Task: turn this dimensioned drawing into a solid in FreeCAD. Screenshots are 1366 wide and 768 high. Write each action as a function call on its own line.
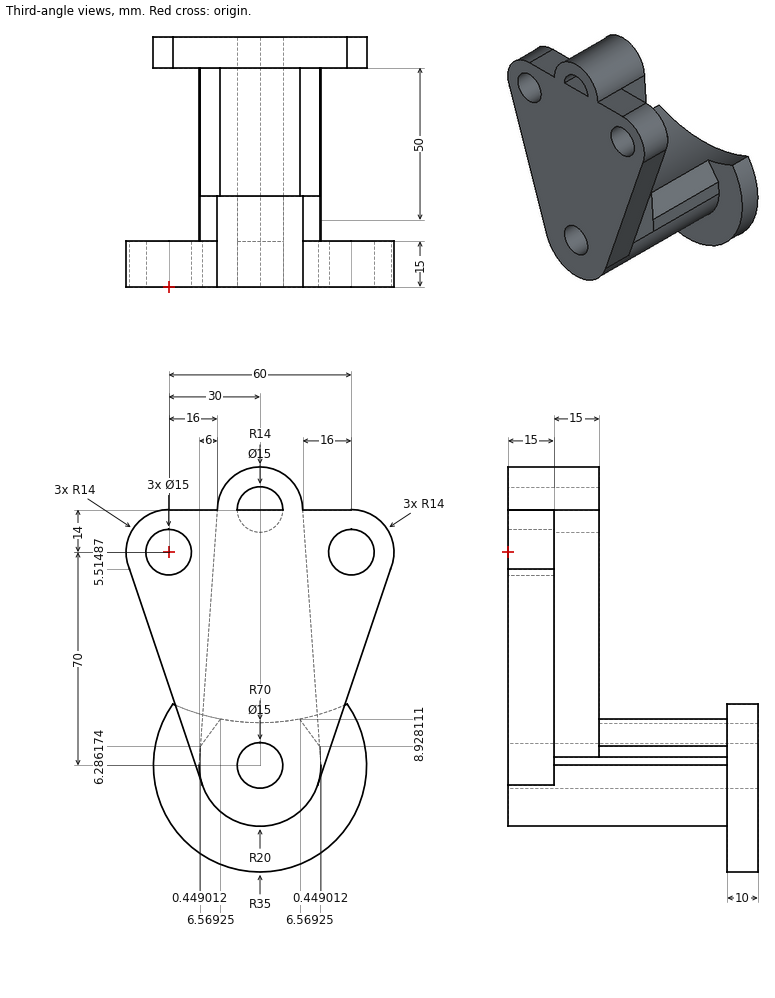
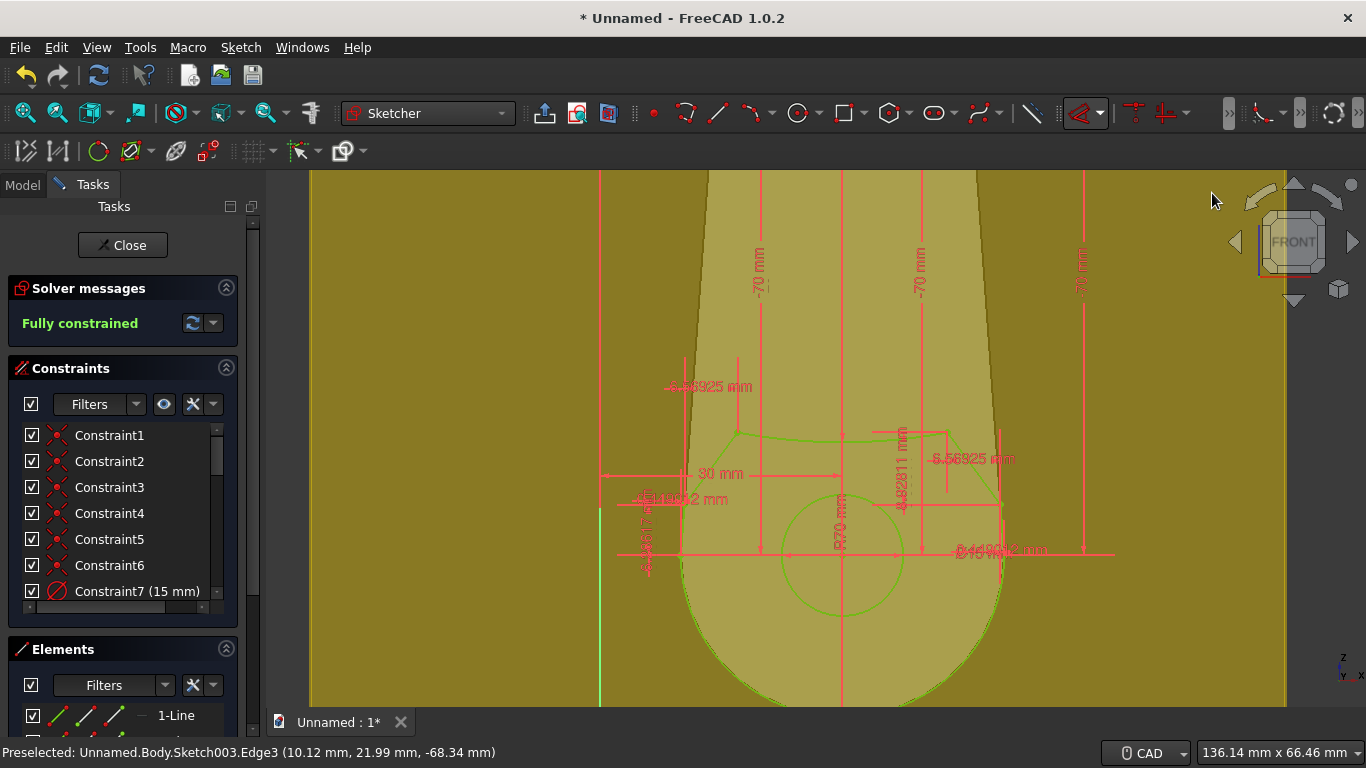
click(123, 245)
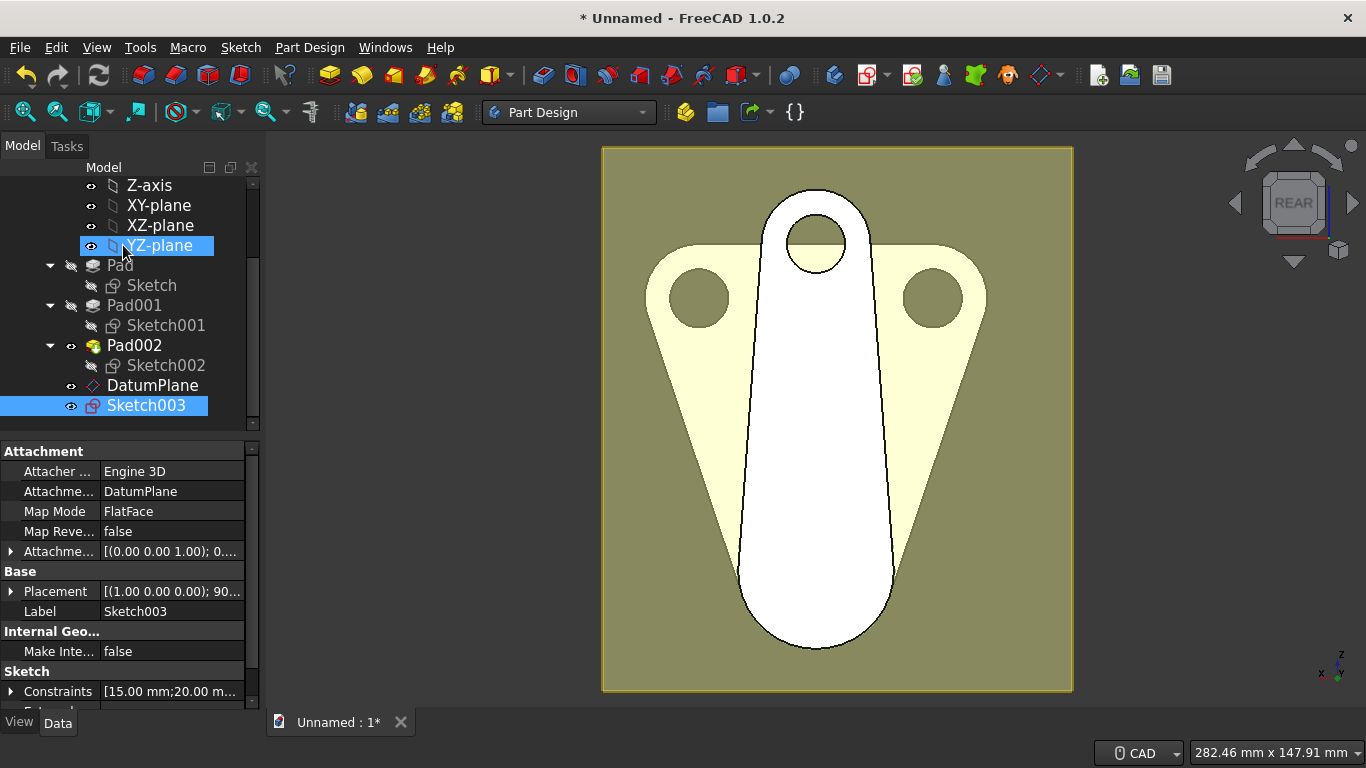
click(330, 76)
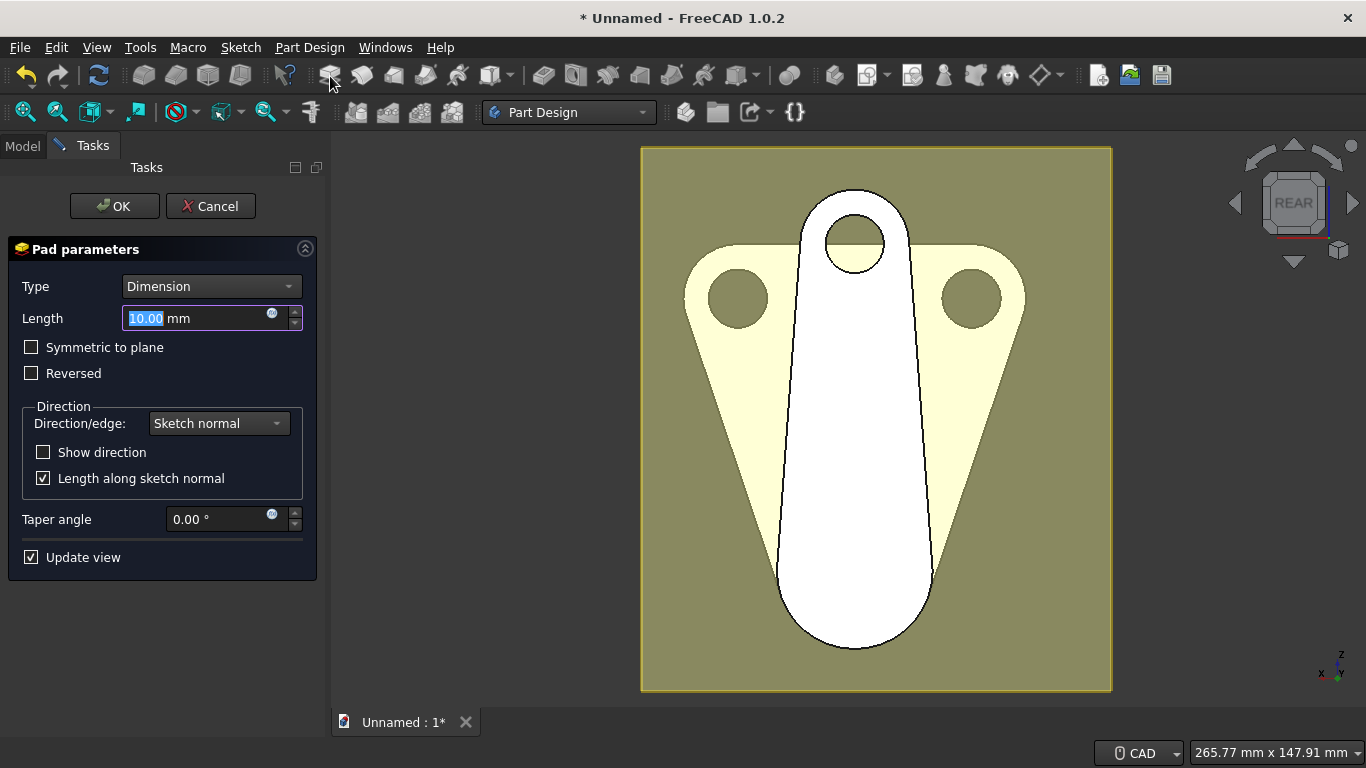
text(50)
key(Tab)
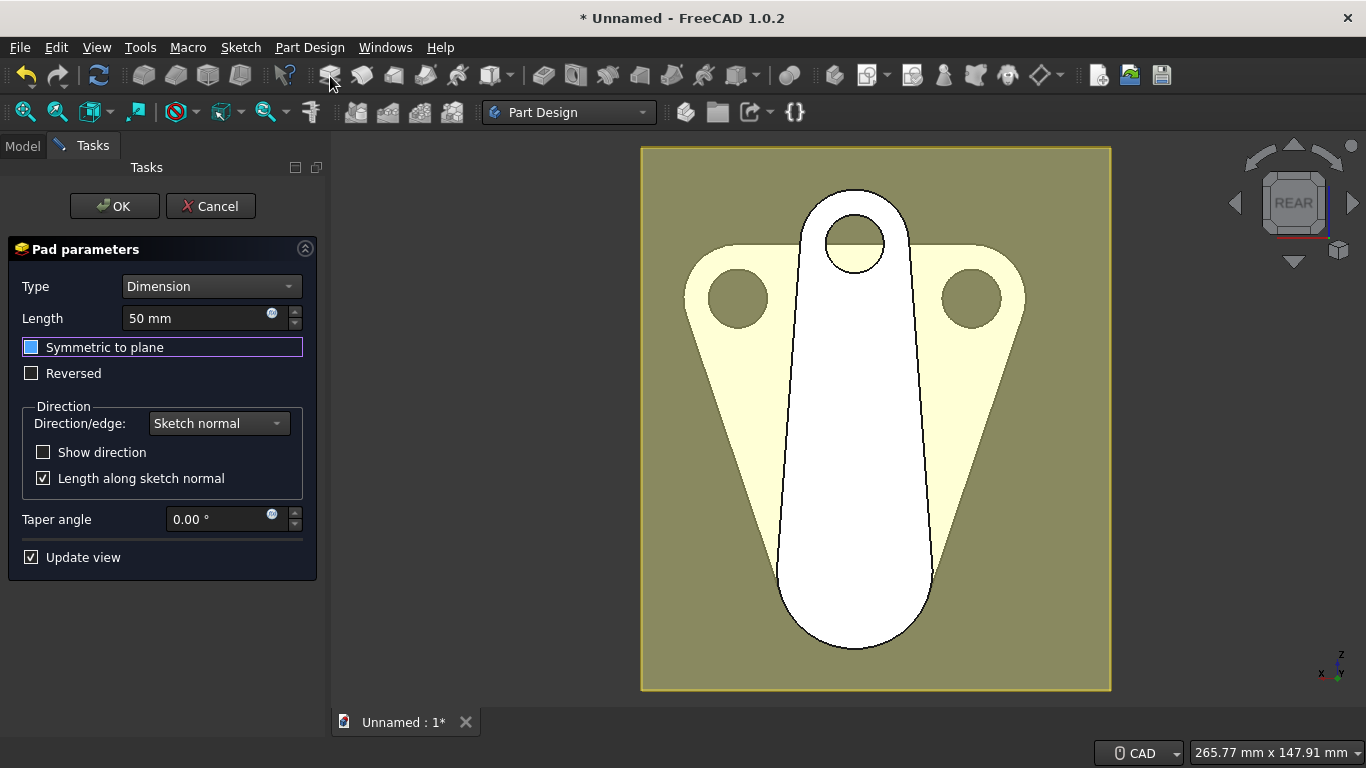
click(30, 373)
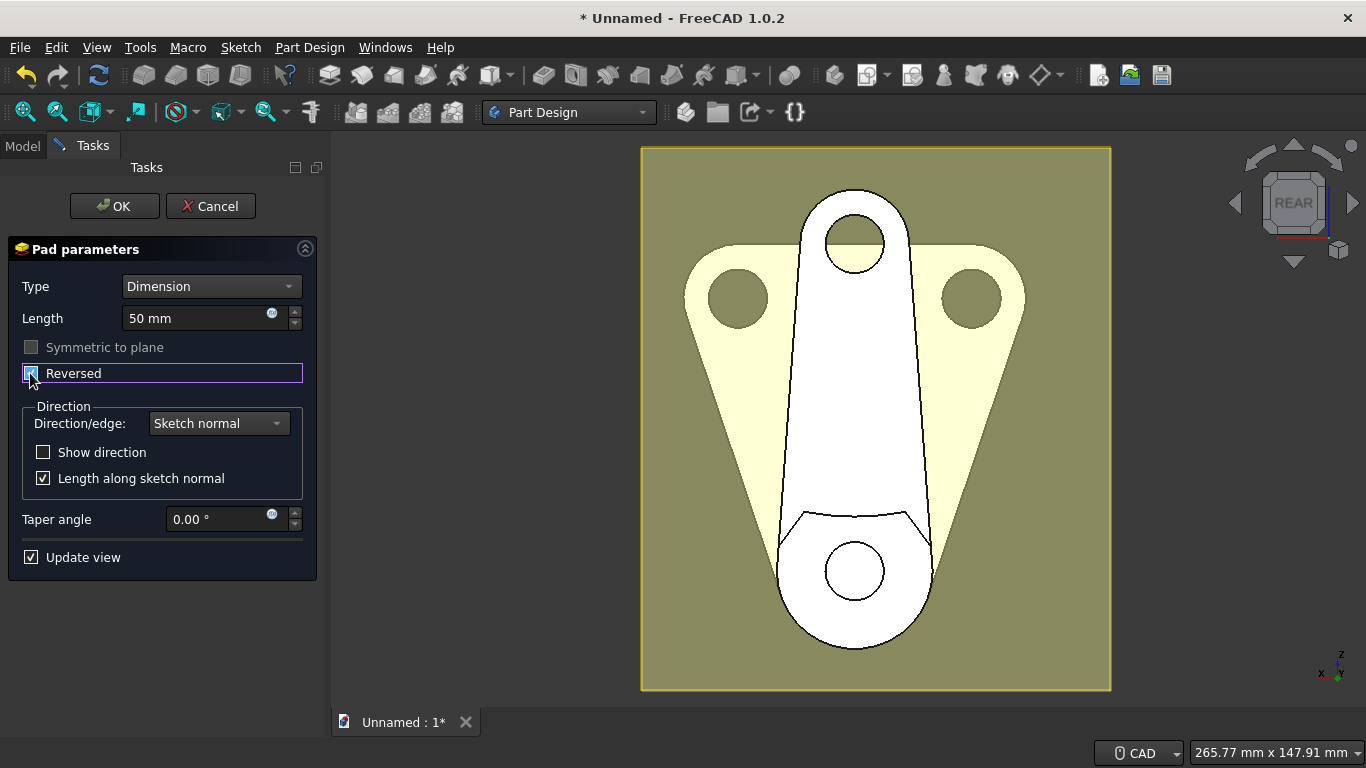
click(115, 206)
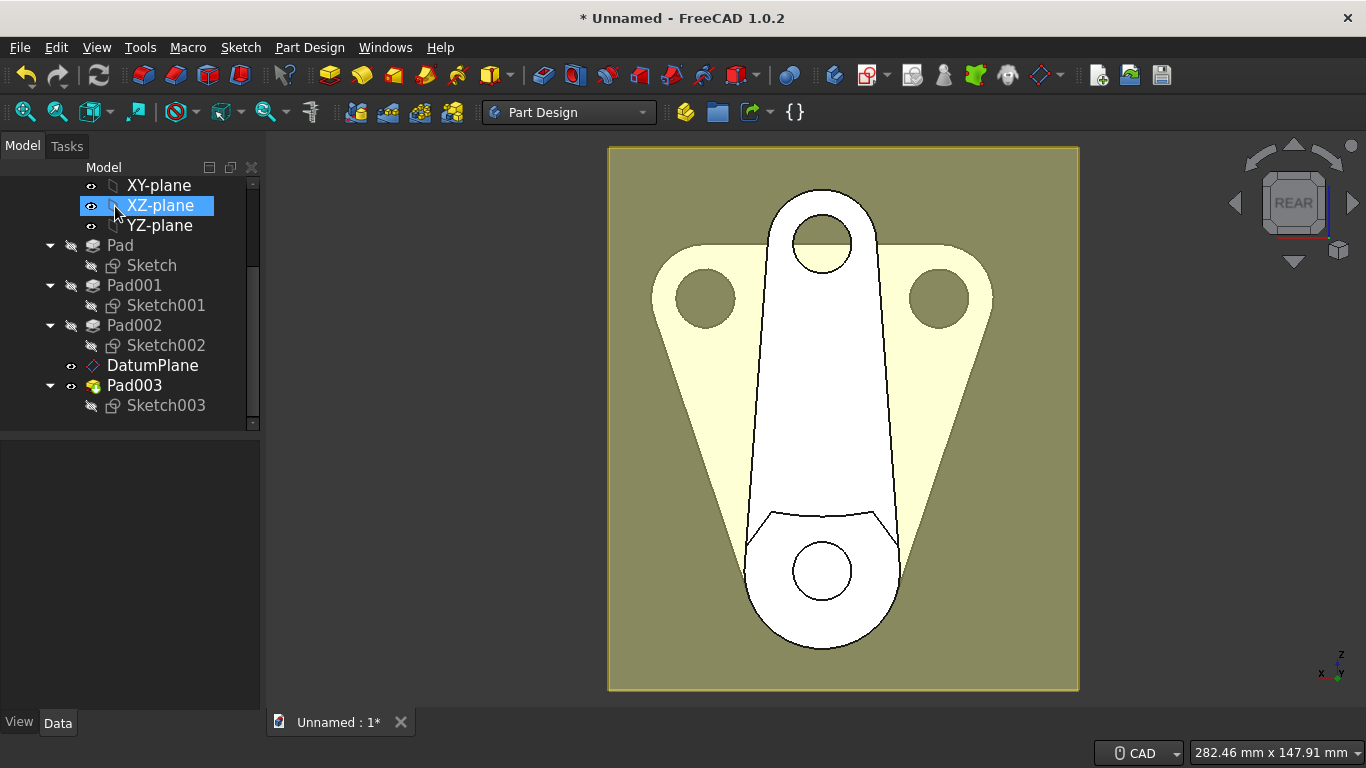
click(116, 366)
key(space)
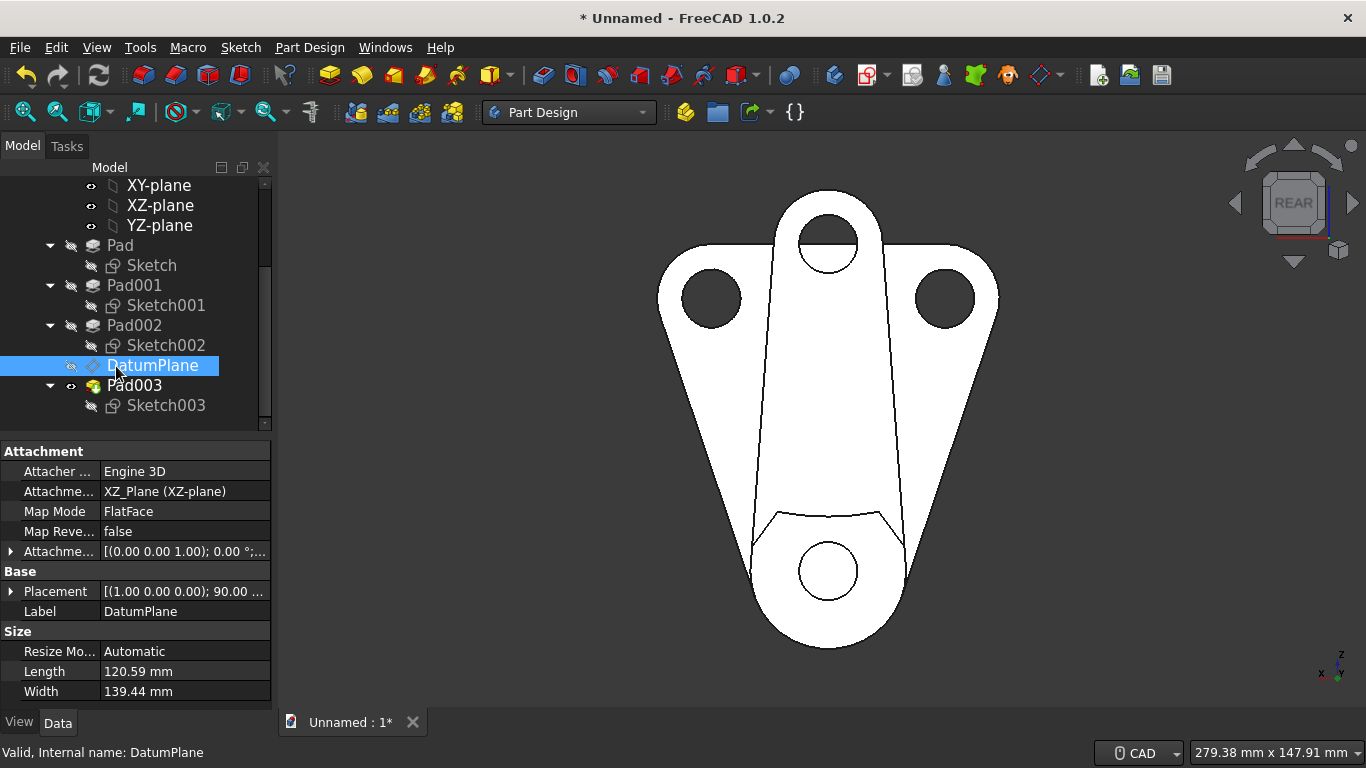
click(806, 619)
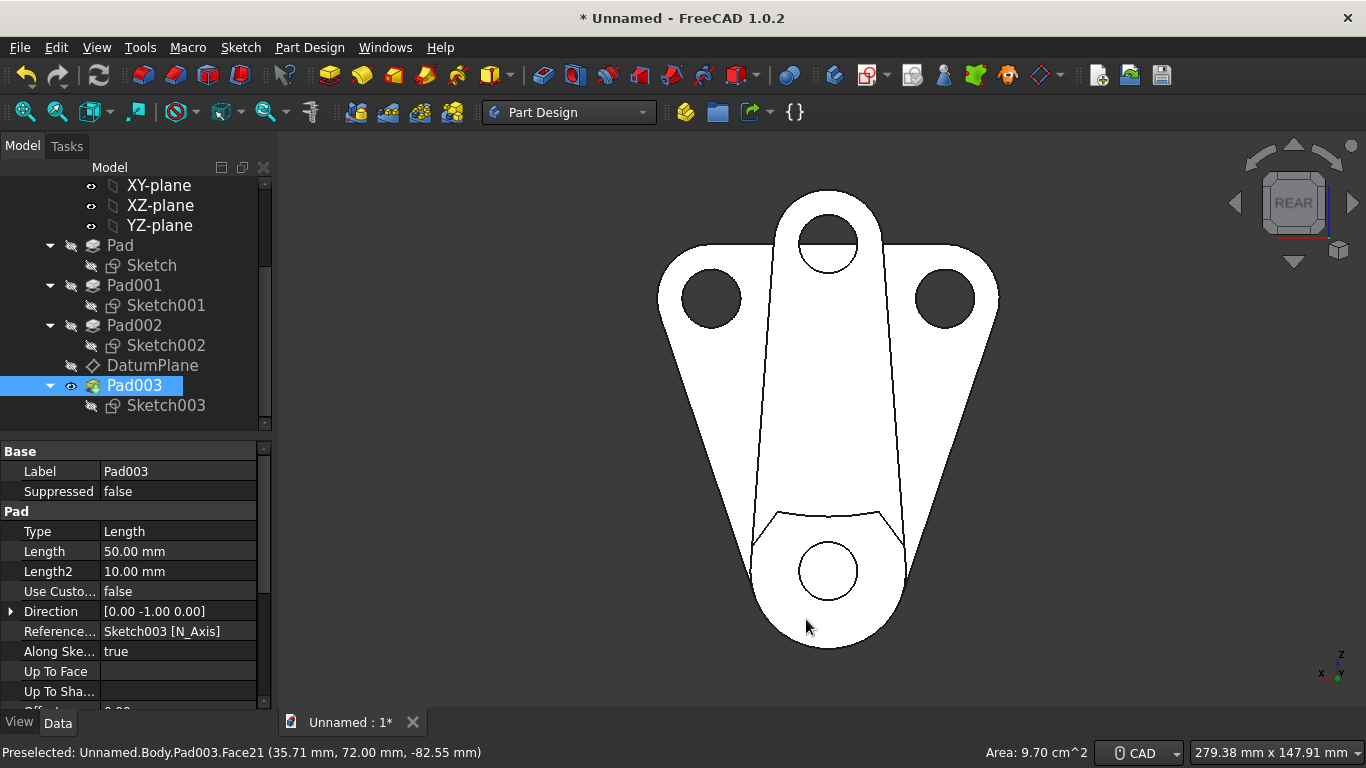
click(868, 76)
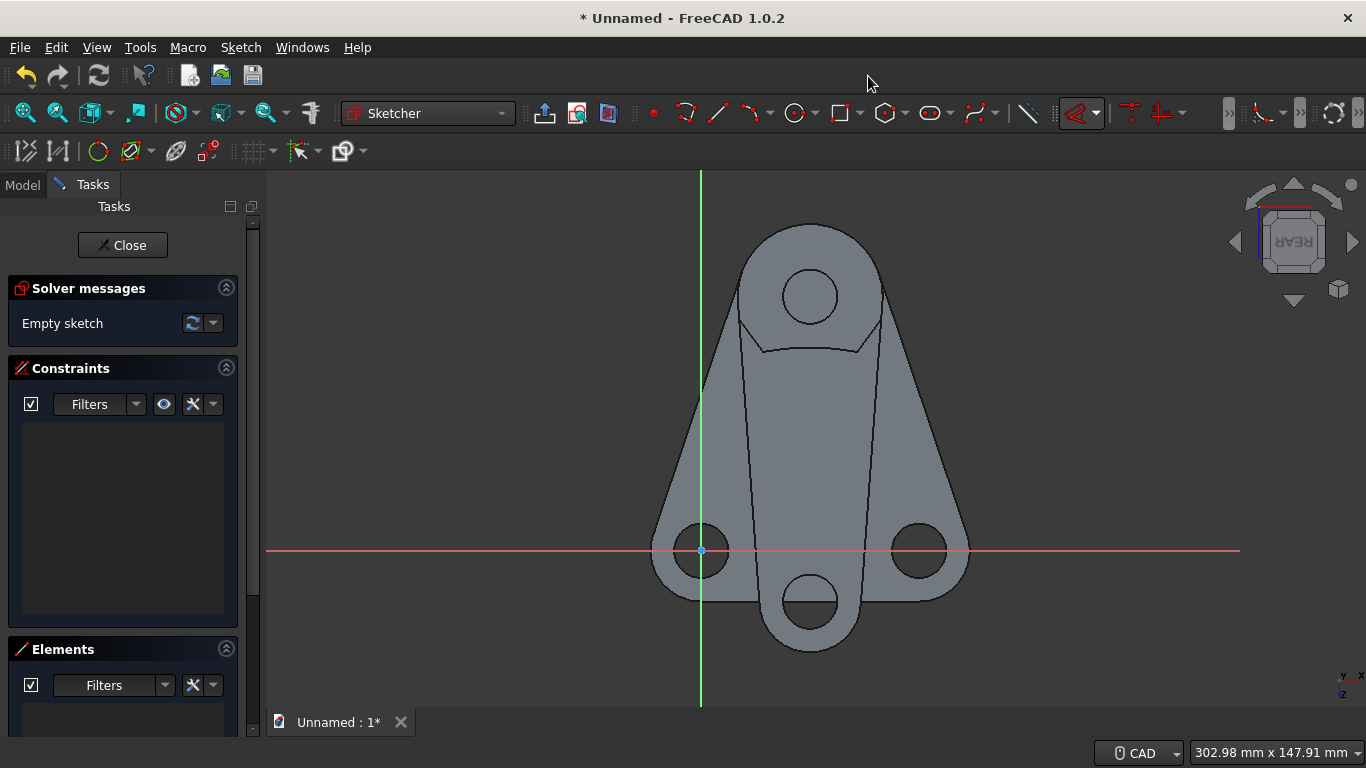
scroll(476, 679, down, 1)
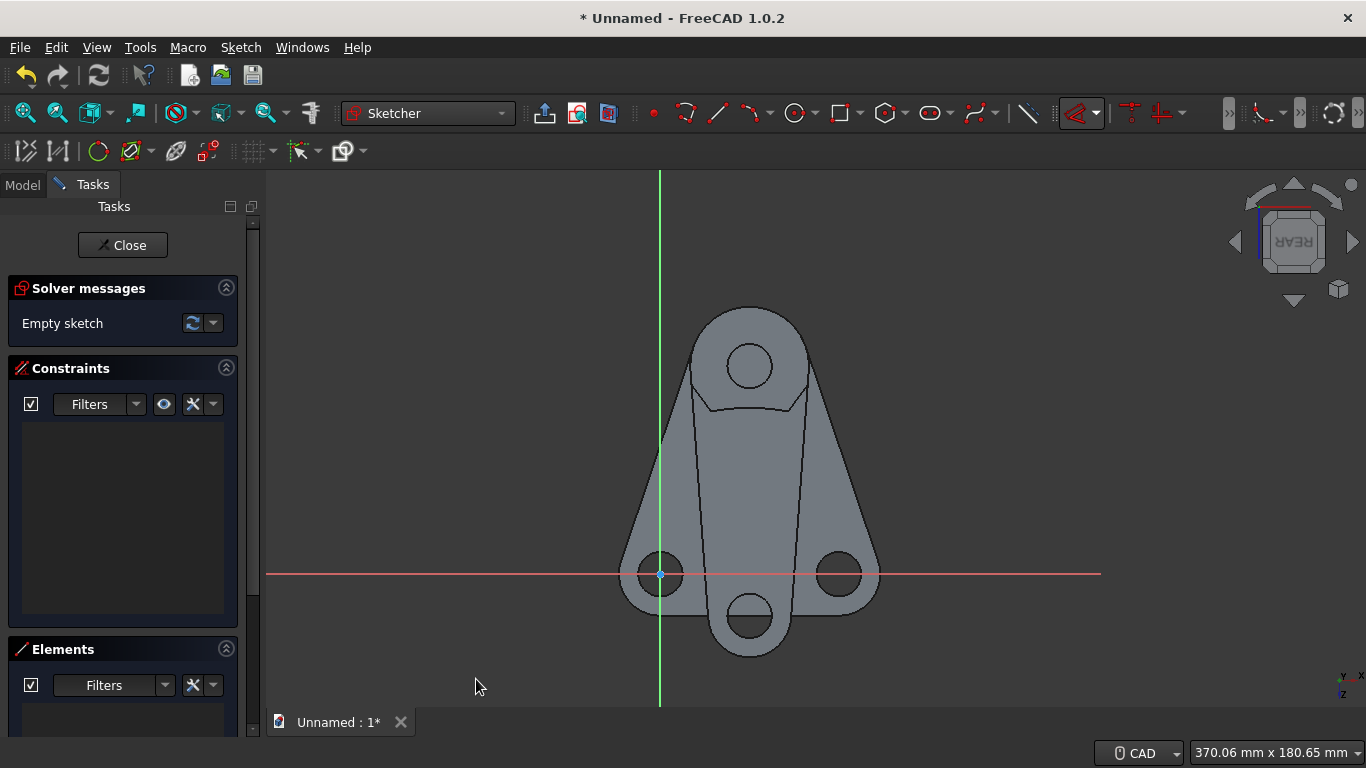
click(750, 114)